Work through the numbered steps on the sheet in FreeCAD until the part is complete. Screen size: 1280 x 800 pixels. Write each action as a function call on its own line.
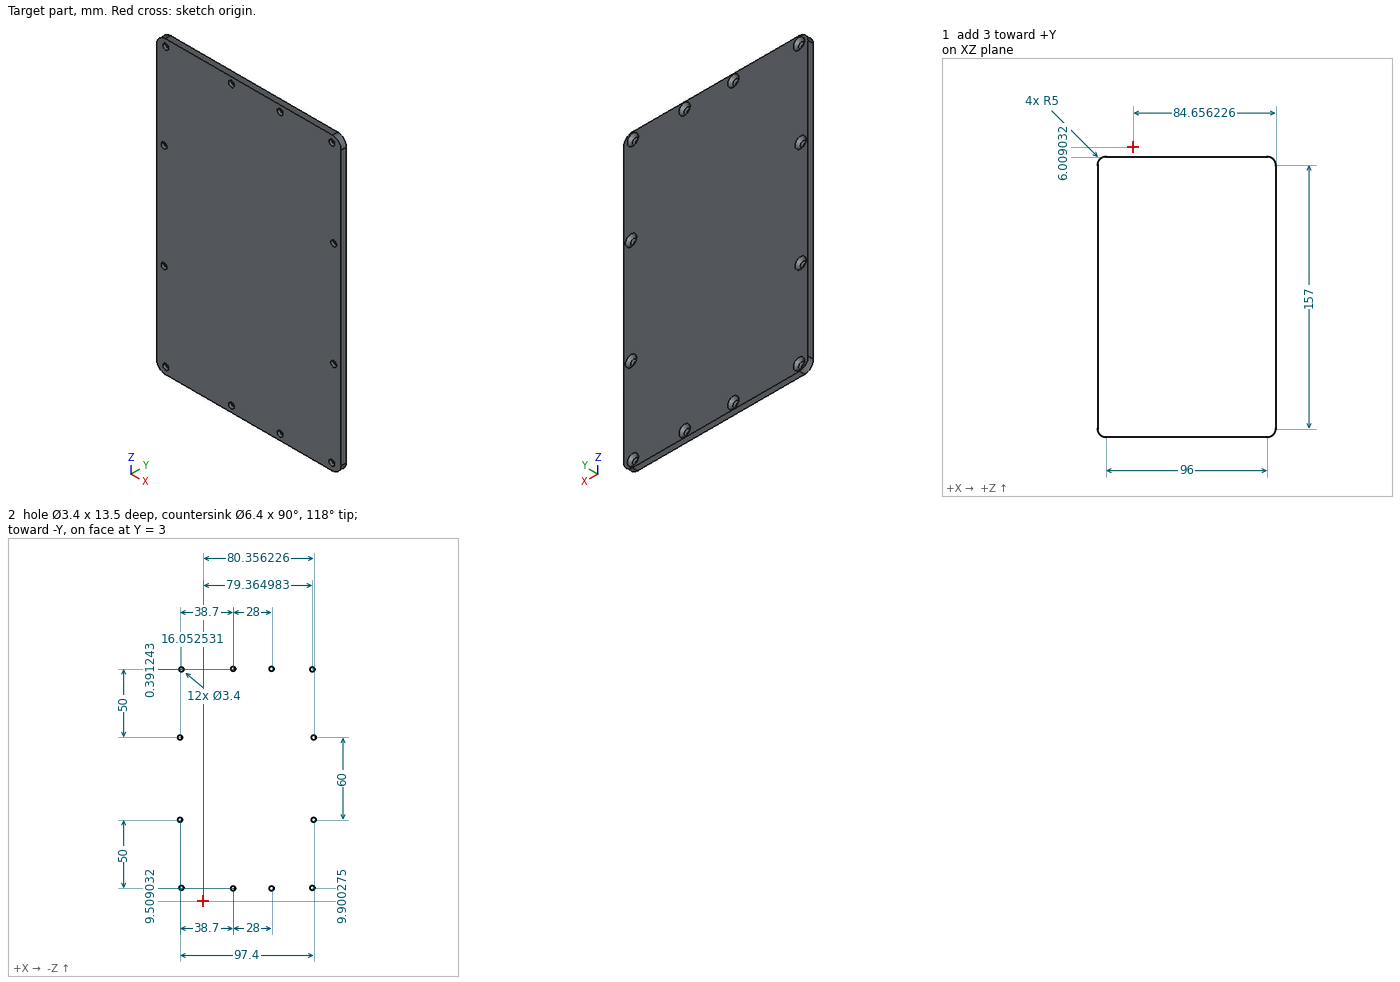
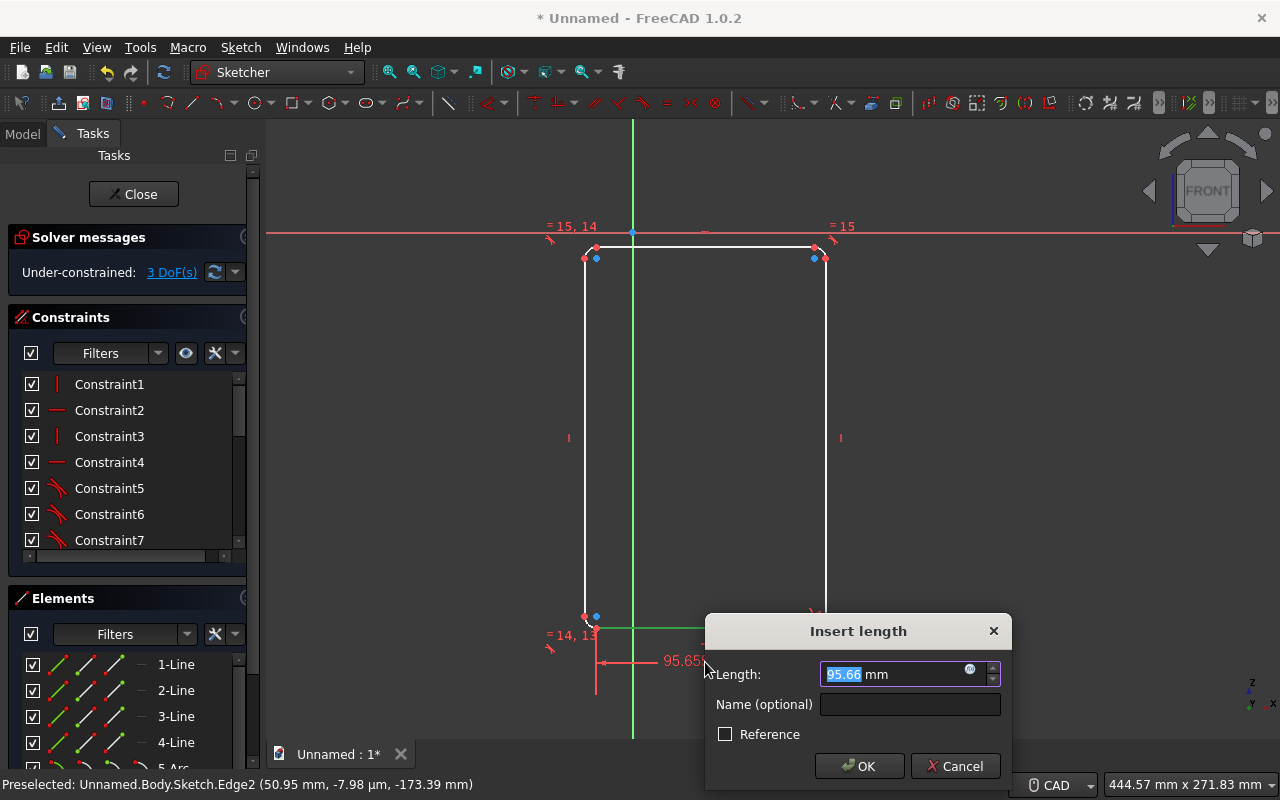
text(96)
key(Return)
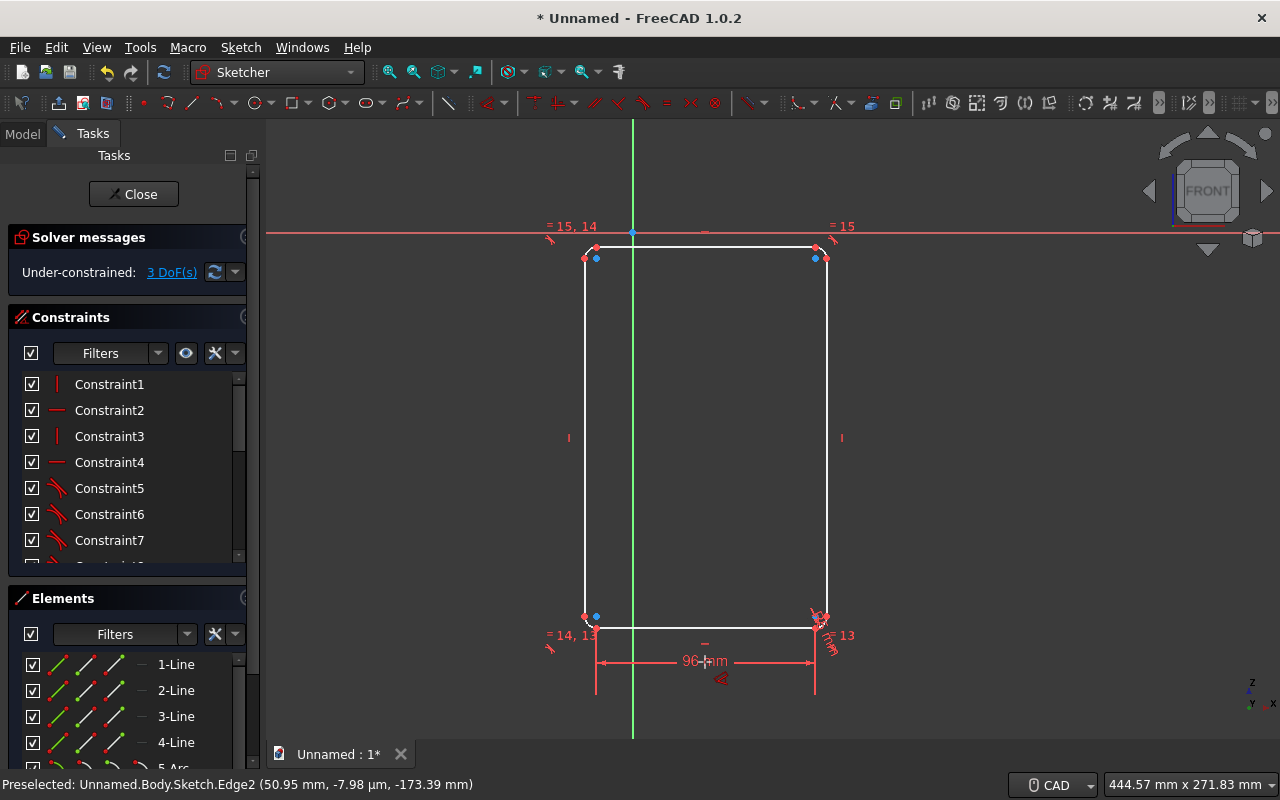
click(827, 366)
click(861, 438)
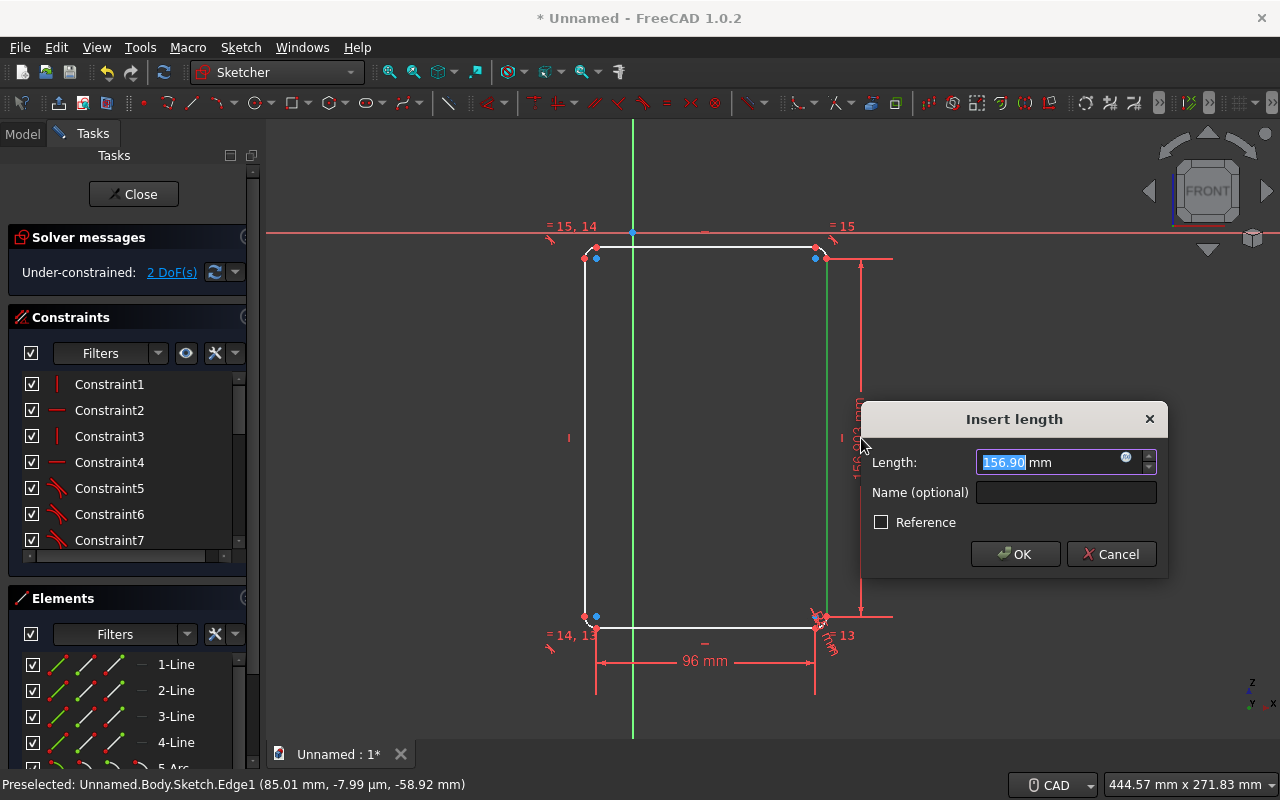
text(157)
key(Return)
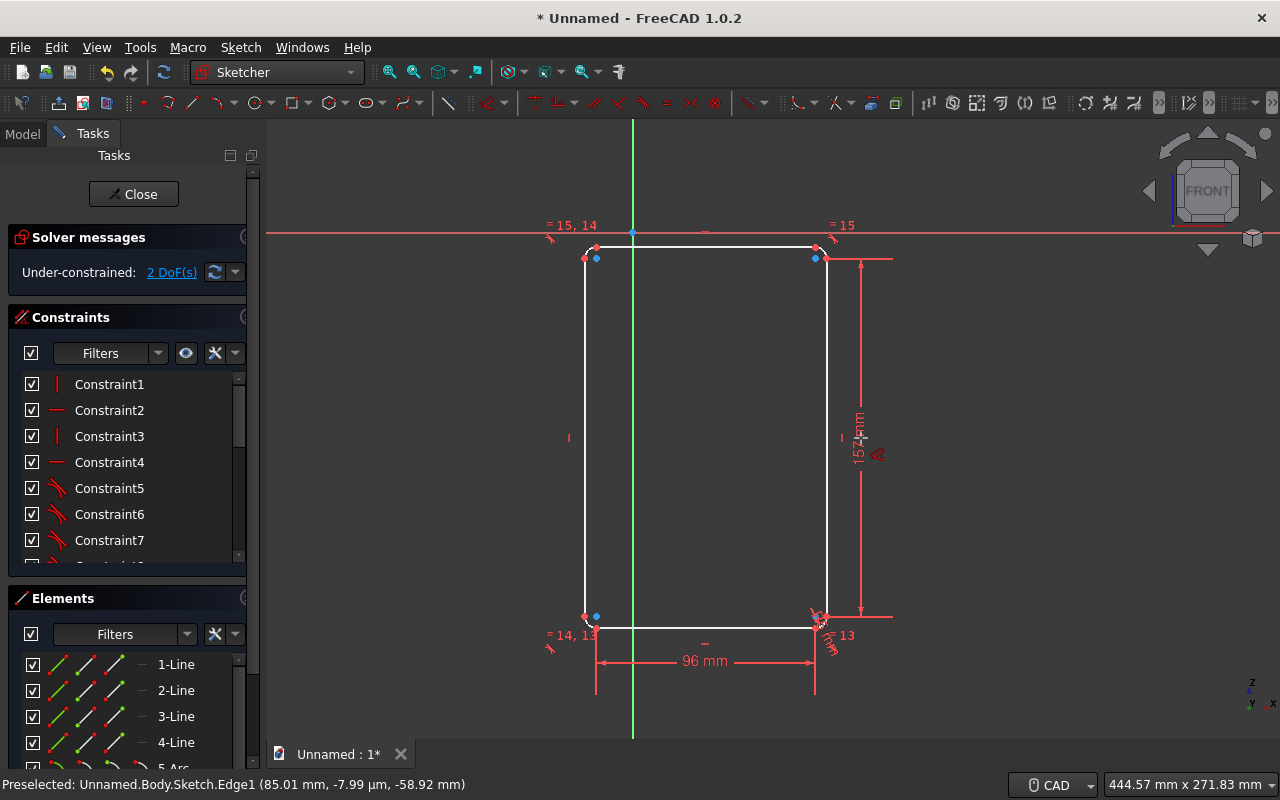
scroll(596, 247, up, 6)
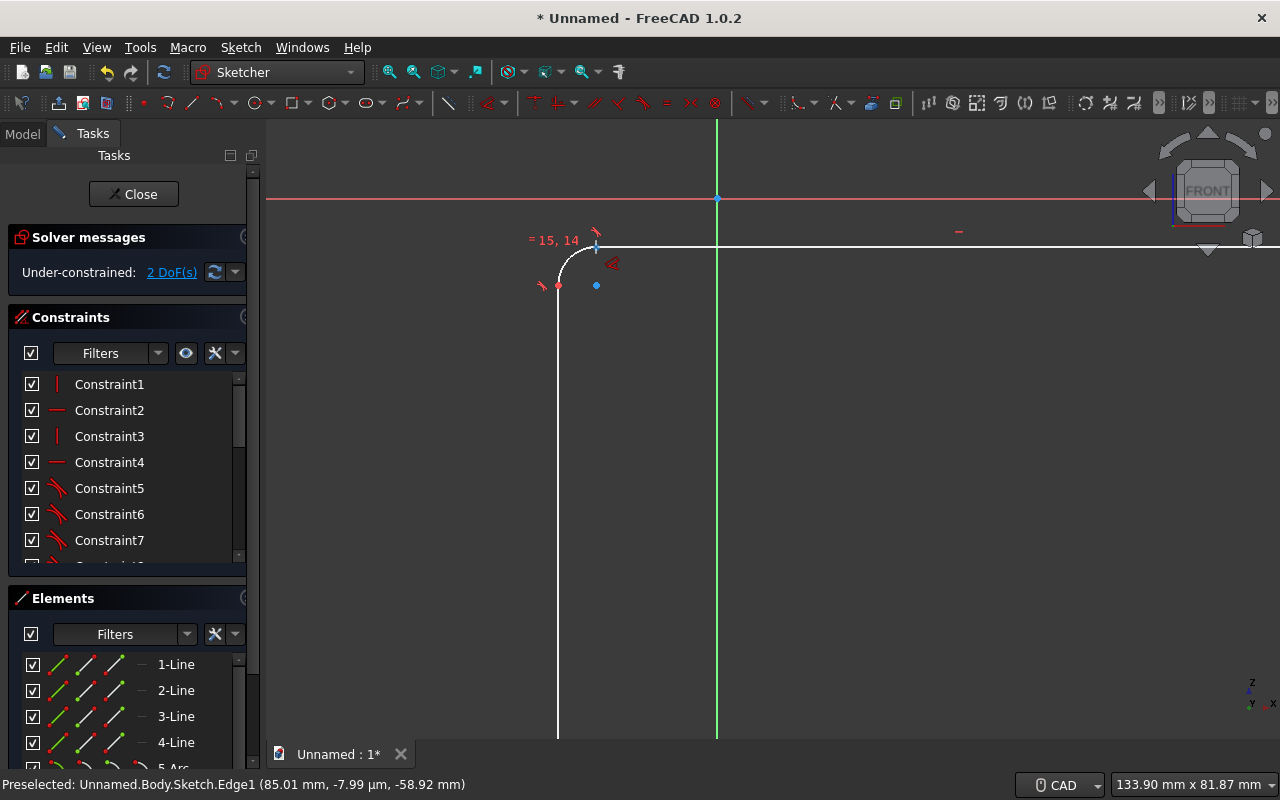
click(596, 247)
click(562, 223)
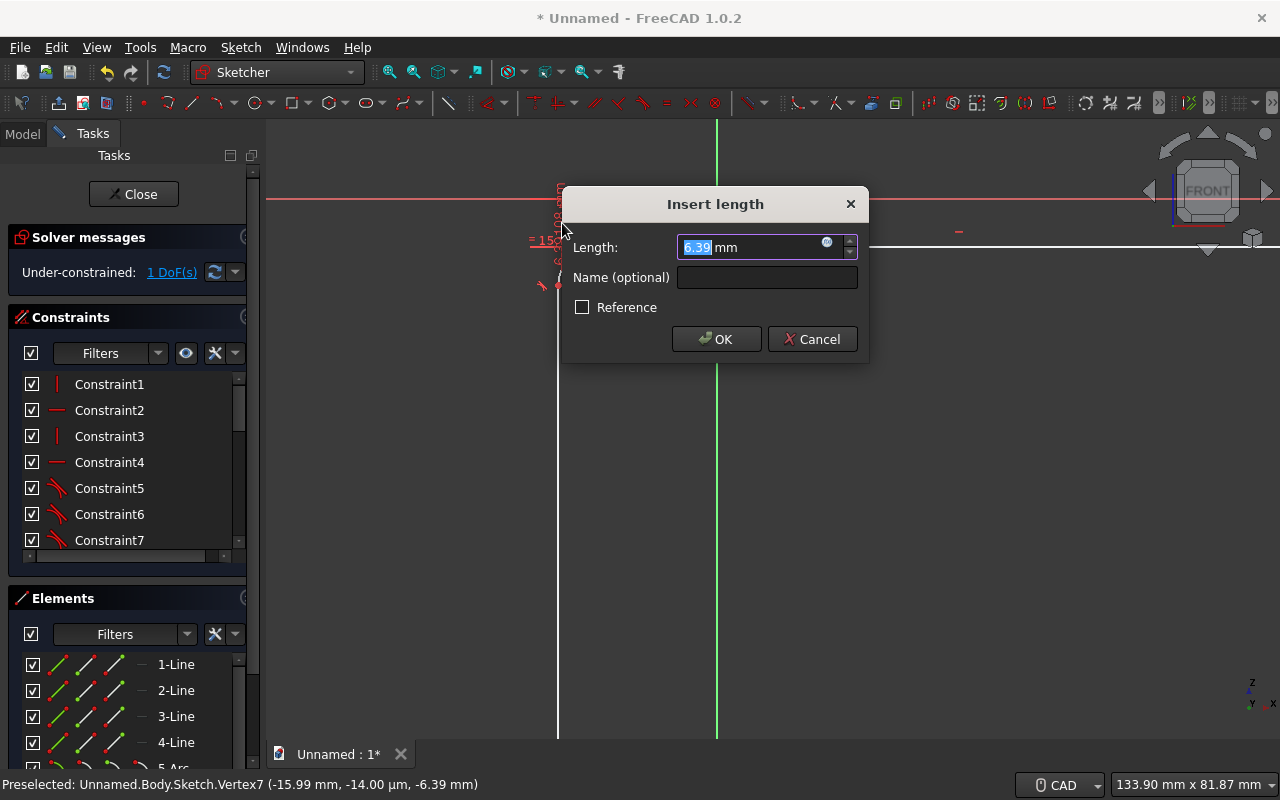
text(6.009032)
key(Return)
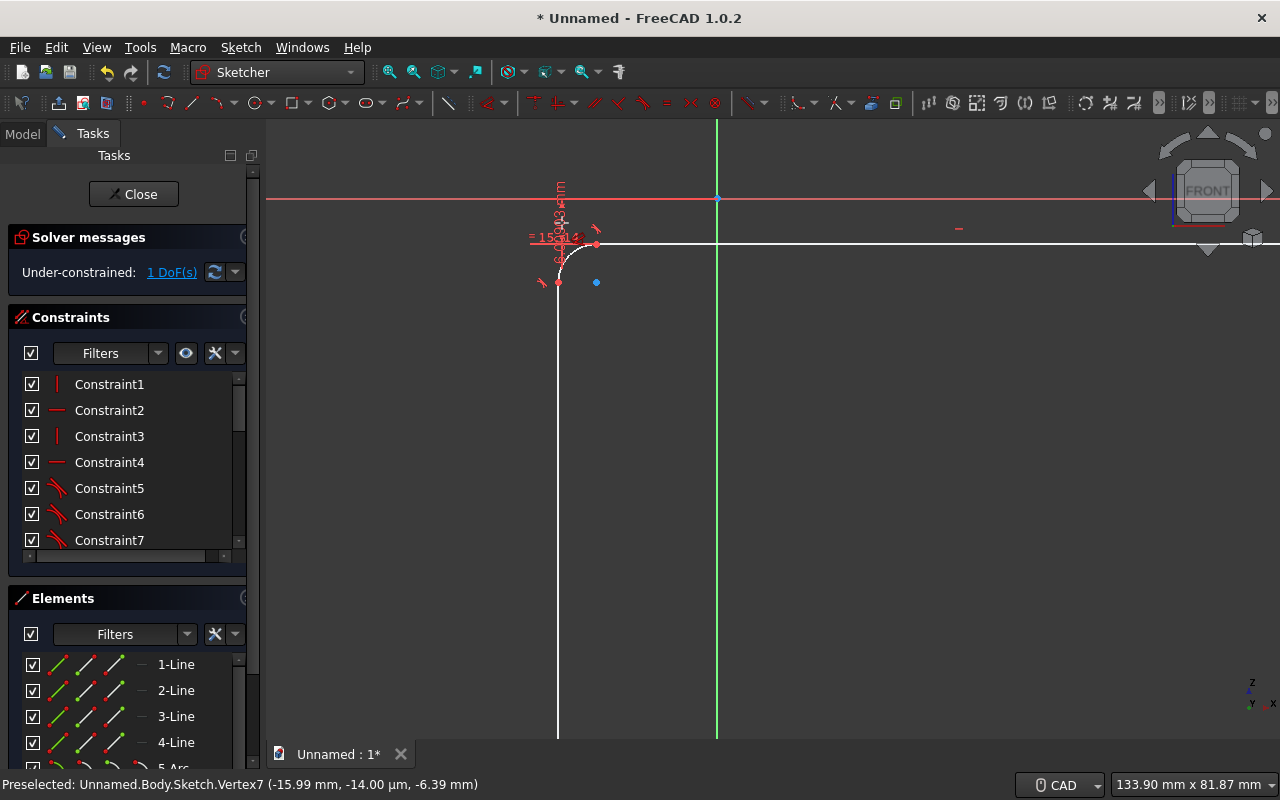
scroll(596, 246, down, 6)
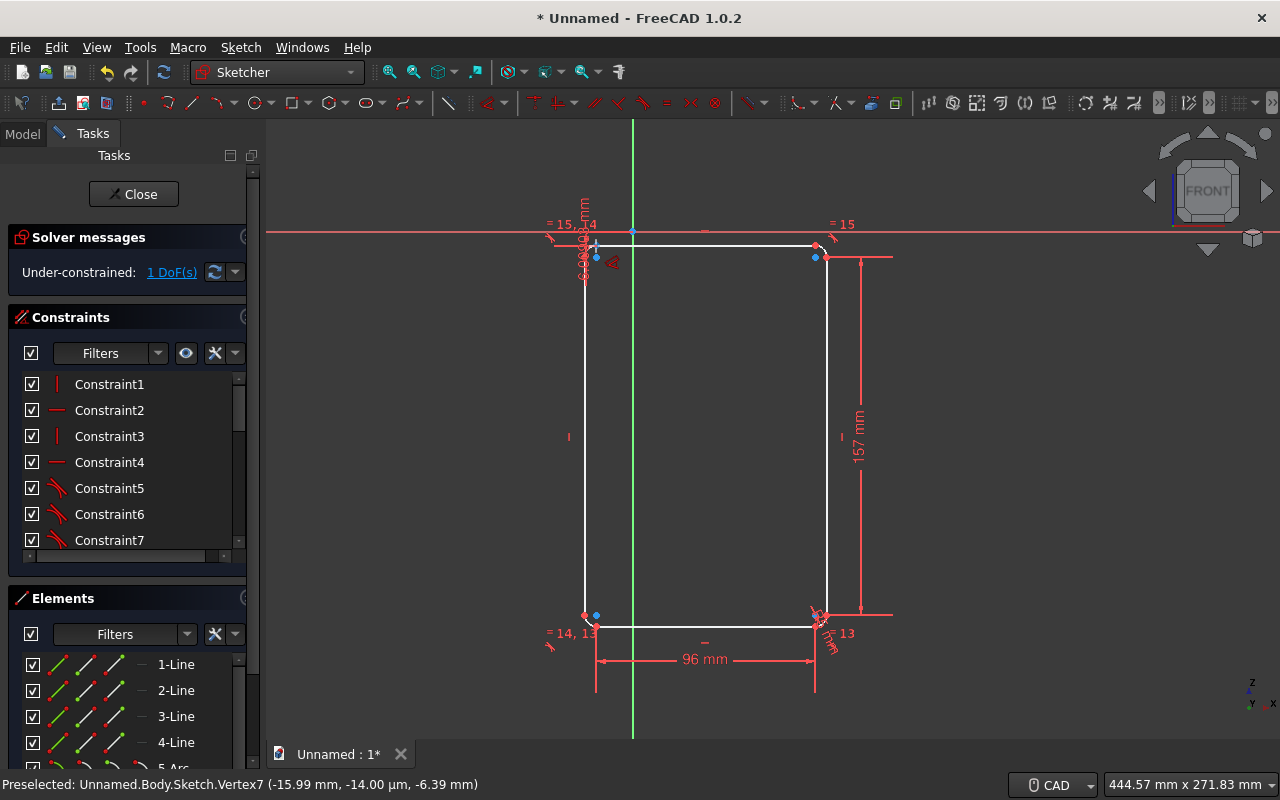
click(827, 257)
click(730, 198)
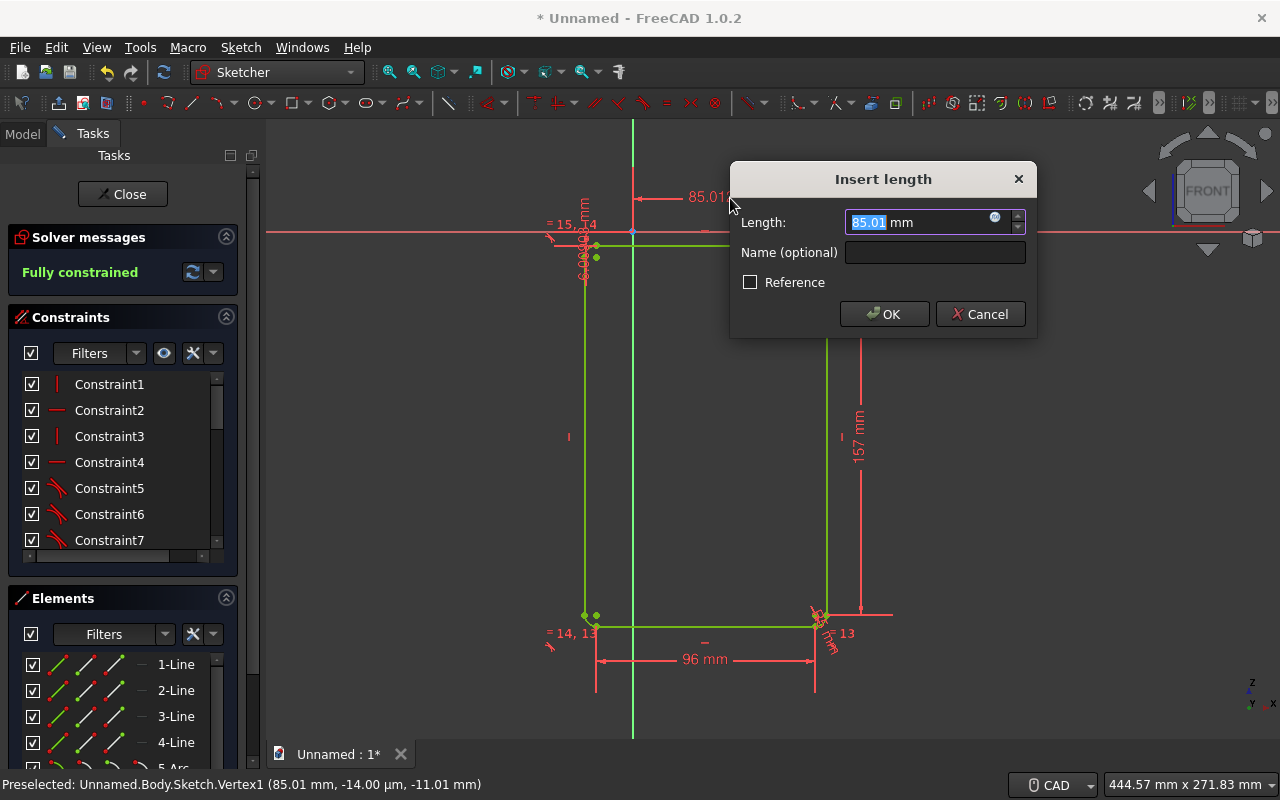
text(84.656226)
key(Return)
key(Escape)